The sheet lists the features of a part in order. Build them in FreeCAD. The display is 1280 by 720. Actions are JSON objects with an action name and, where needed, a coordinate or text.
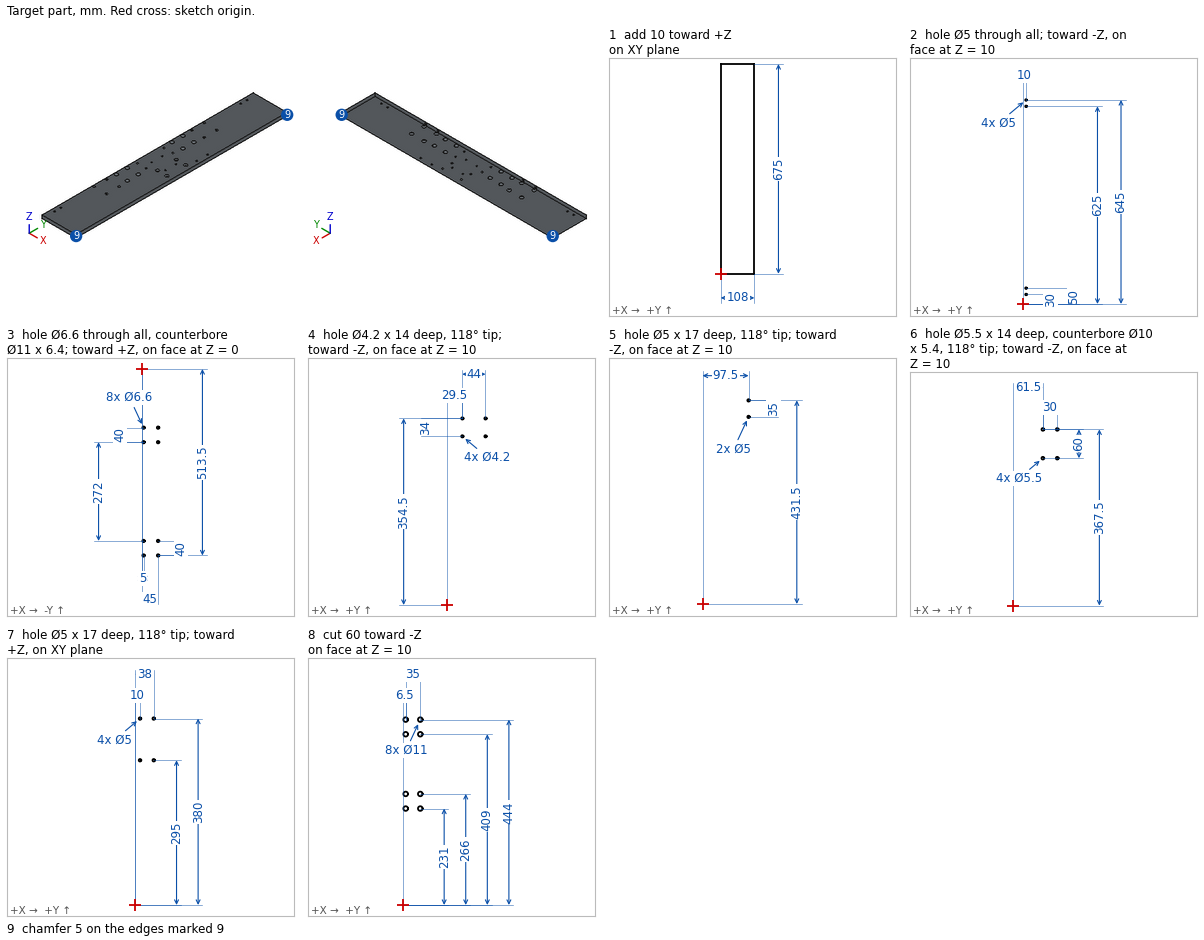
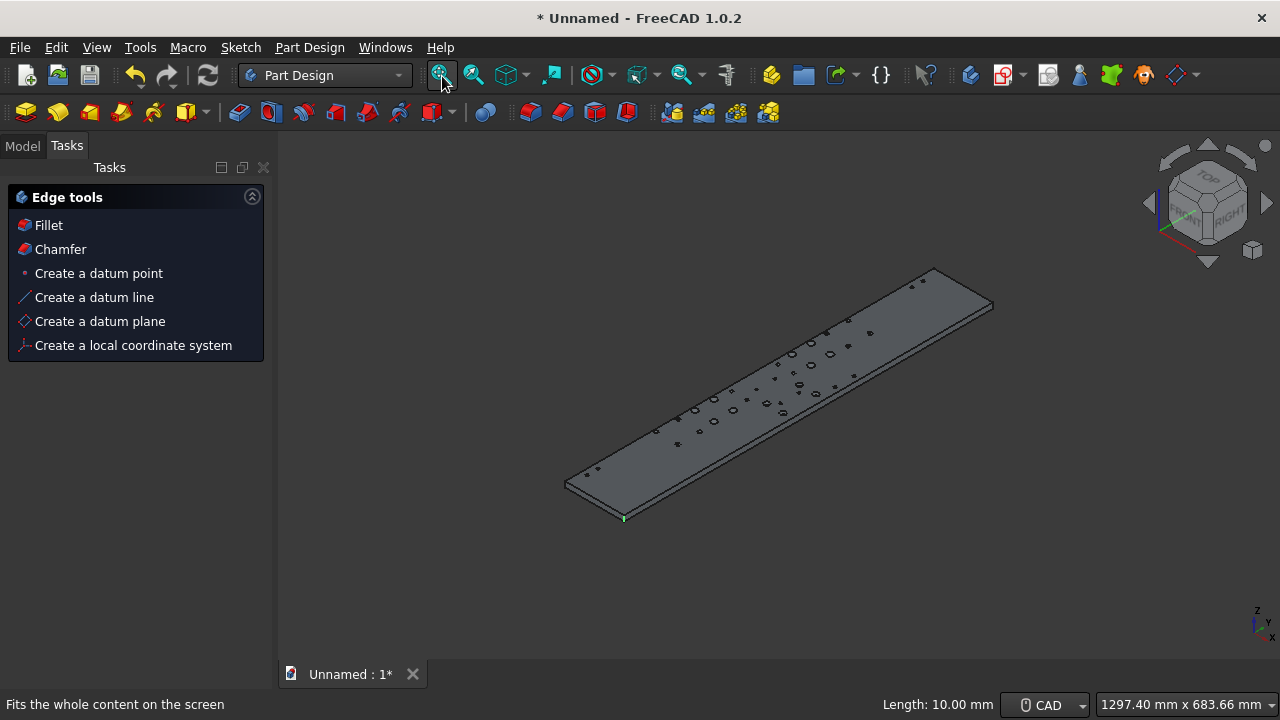
{"action": "scroll", "coordinate": [993, 305], "scroll_direction": "up", "scroll_amount": 9}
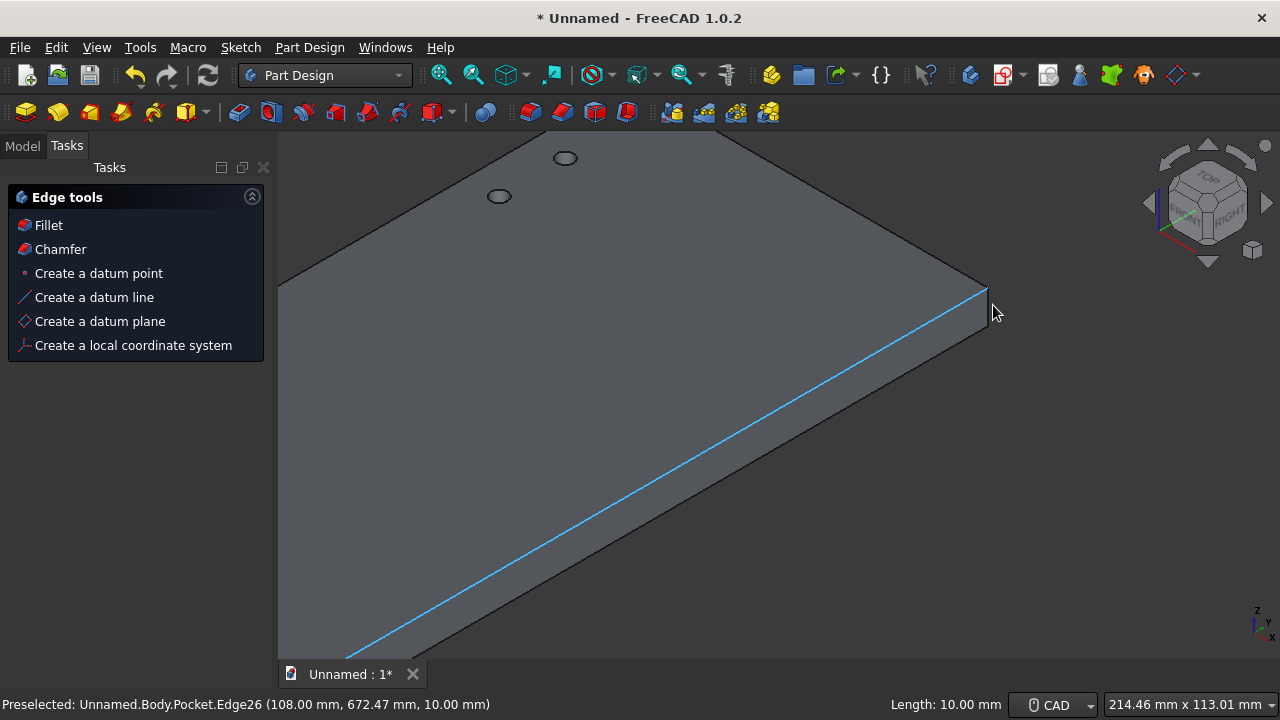
{"action": "left_click", "coordinate": [442, 76]}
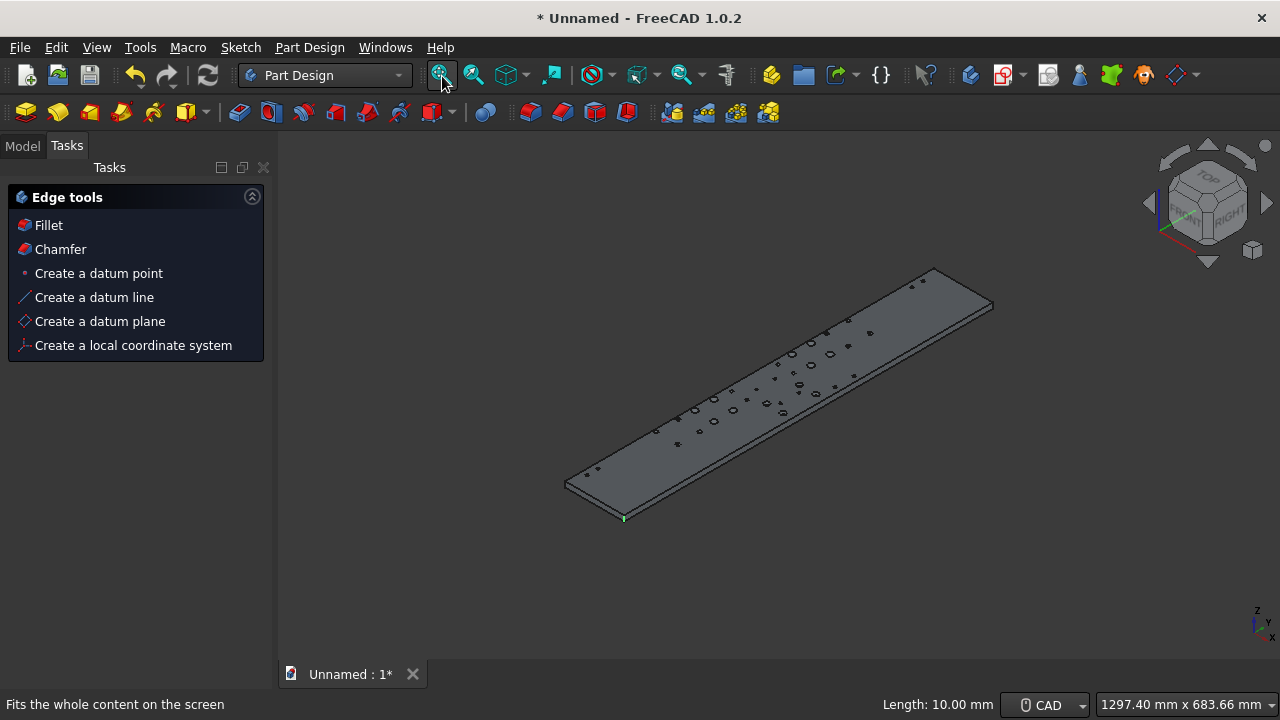
{"action": "key", "text": "1"}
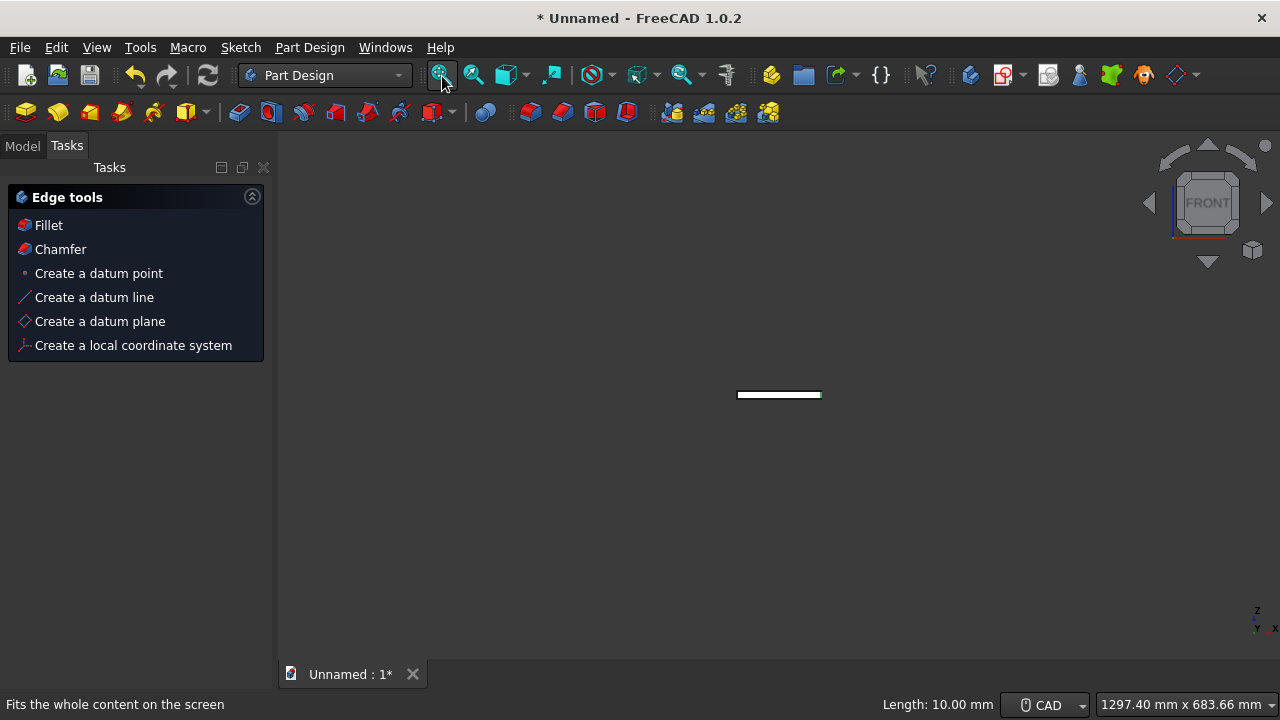
{"action": "left_click", "coordinate": [442, 76]}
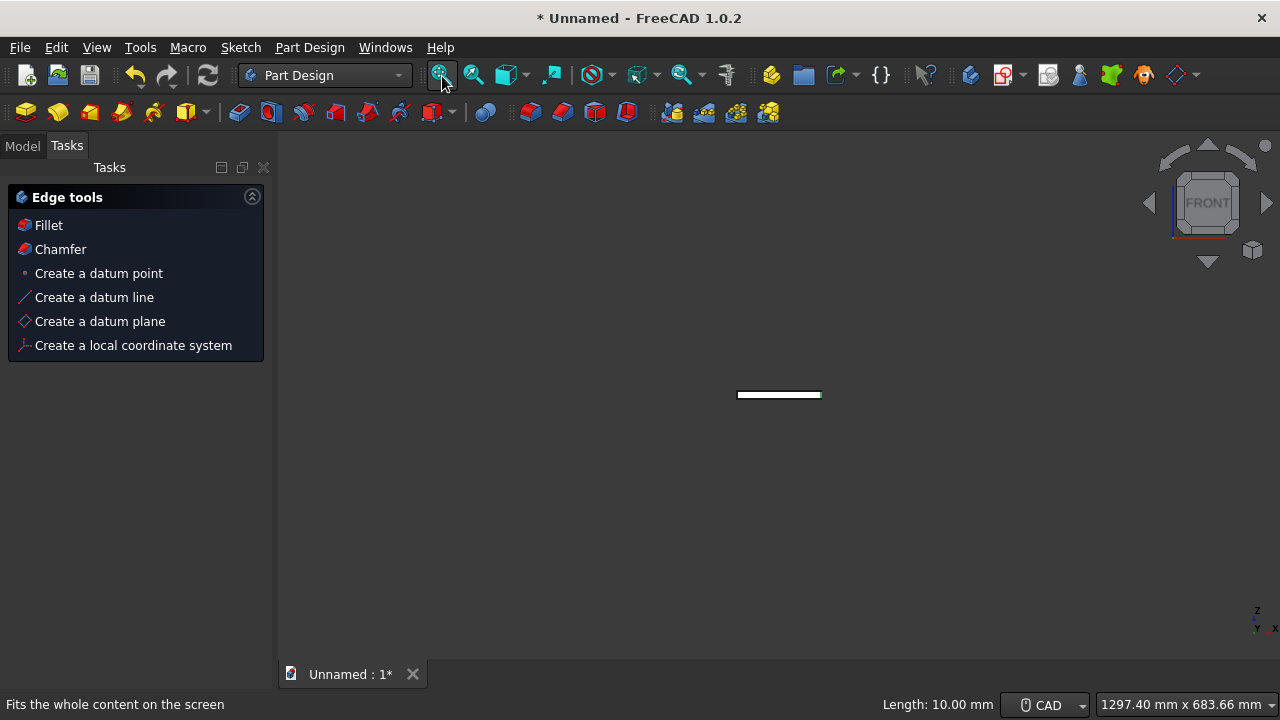
{"action": "scroll", "coordinate": [821, 394], "scroll_direction": "up", "scroll_amount": 9}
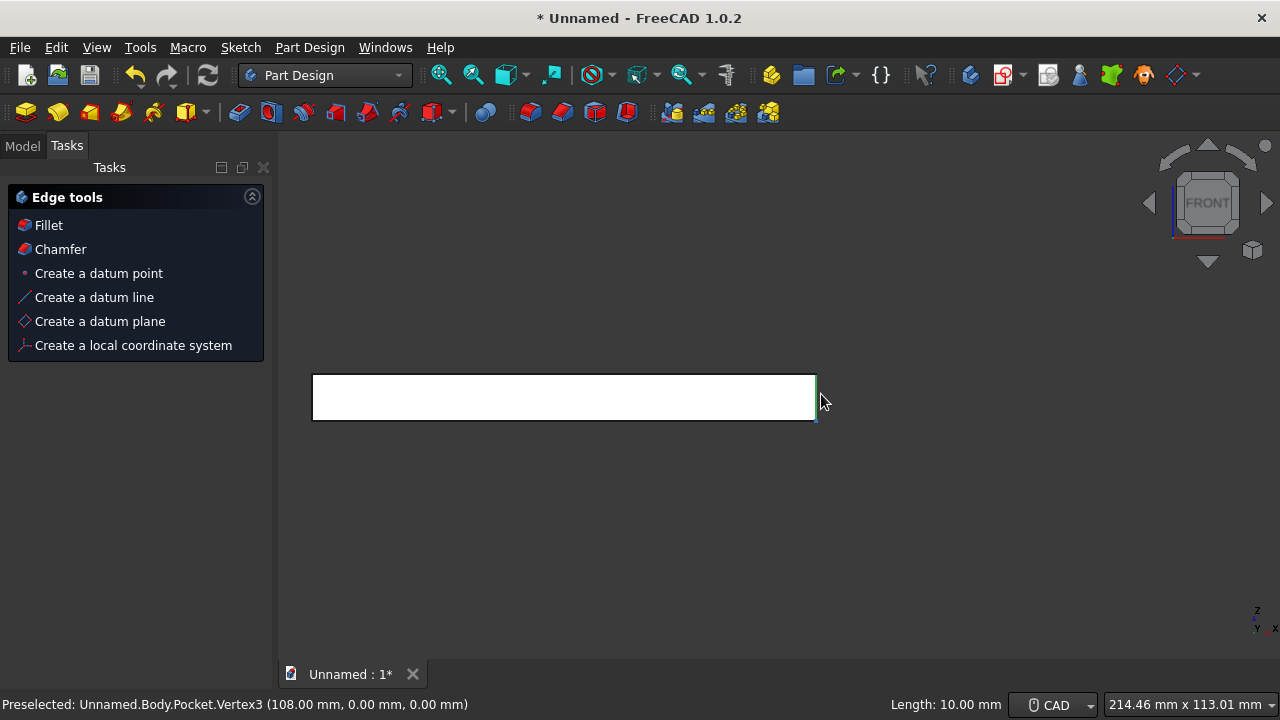
{"action": "left_click", "coordinate": [442, 76]}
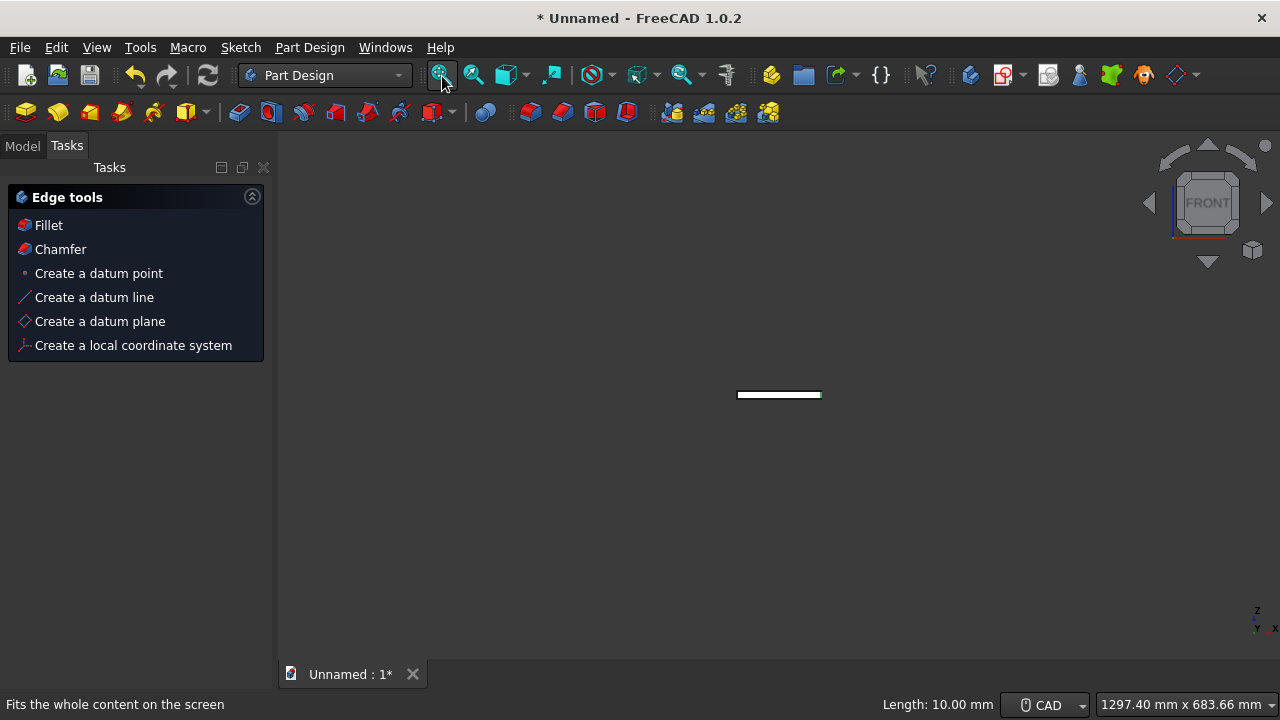
{"action": "key", "text": "3"}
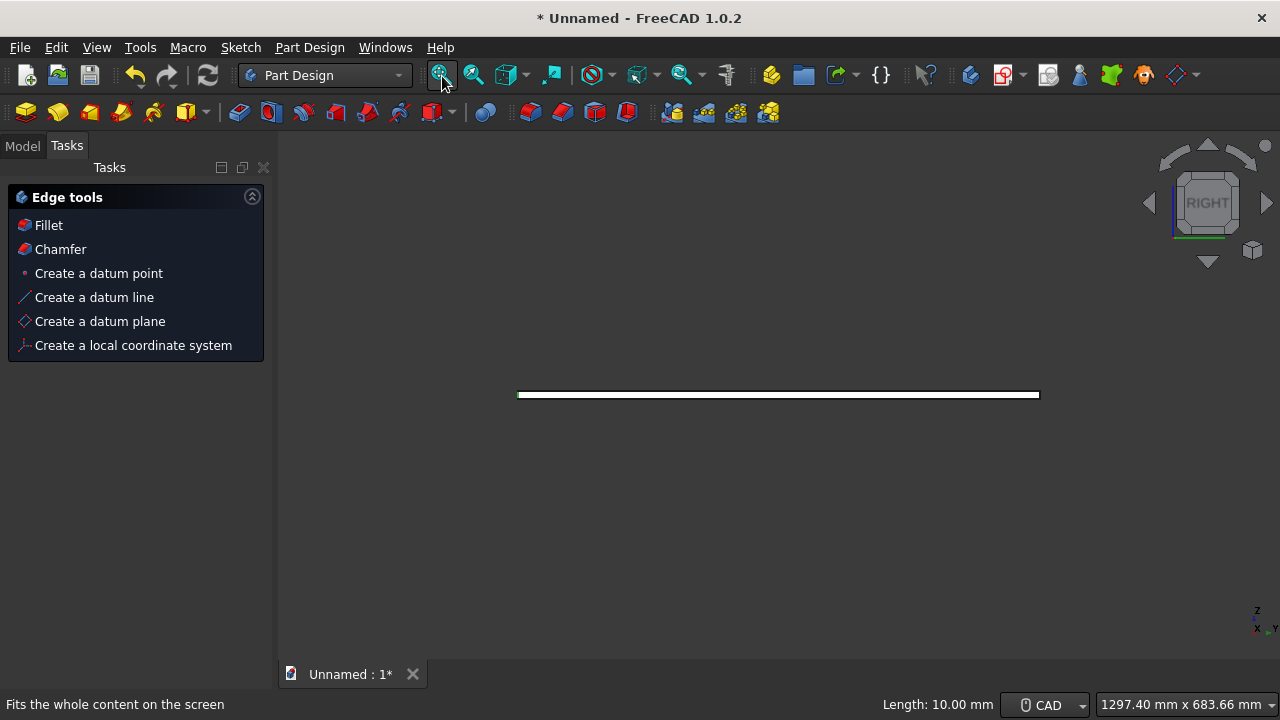
{"action": "scroll", "coordinate": [1040, 394], "scroll_direction": "up", "scroll_amount": 9}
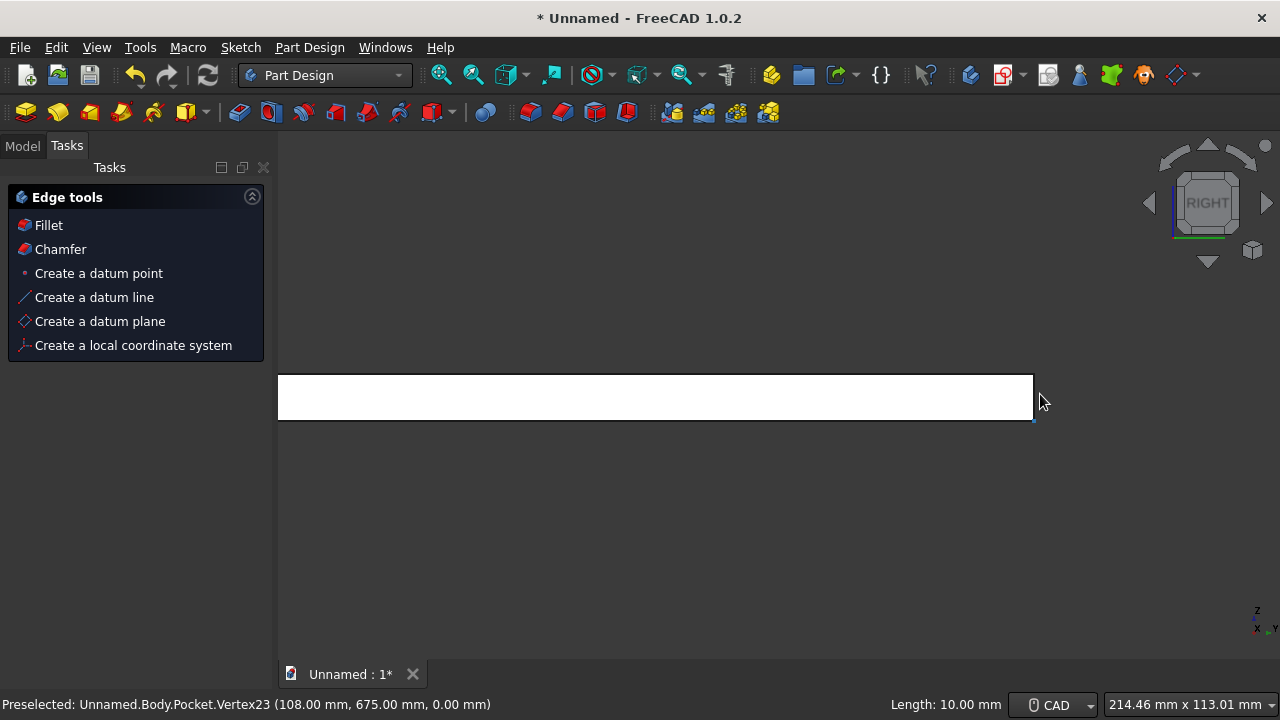
{"action": "left_click", "coordinate": [1034, 397], "text": "ctrl"}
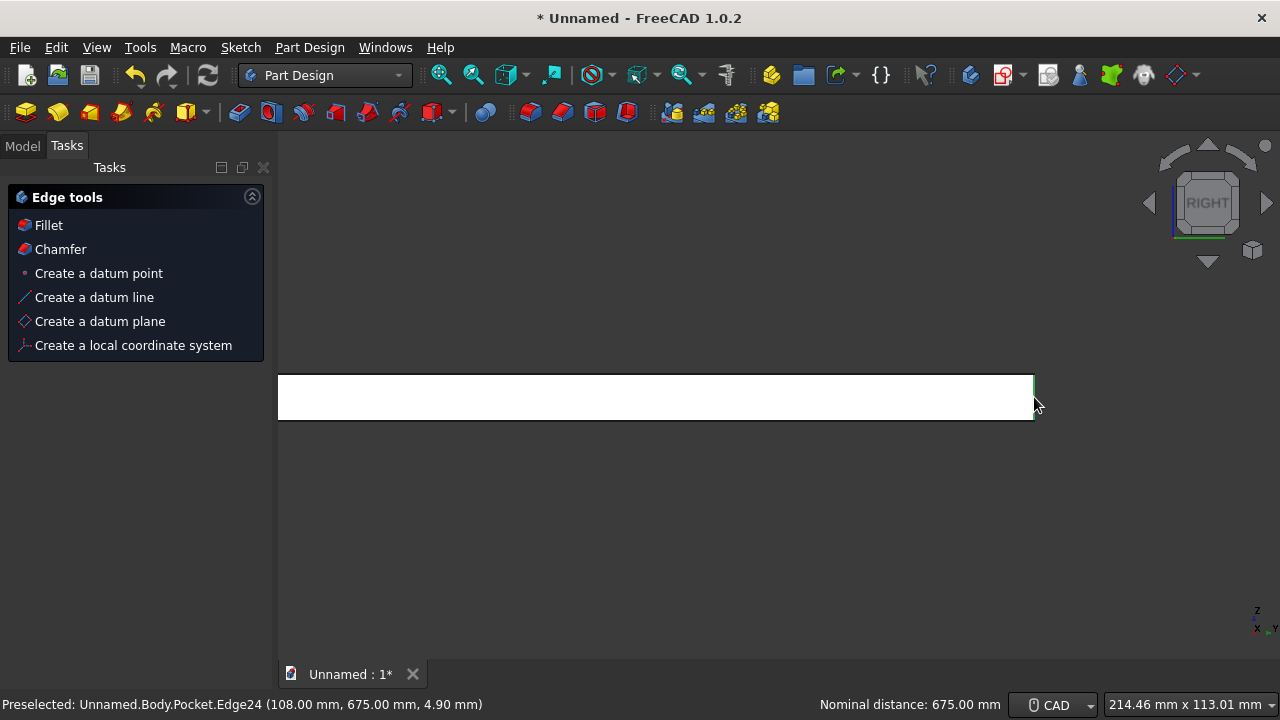
{"action": "left_click", "coordinate": [564, 112]}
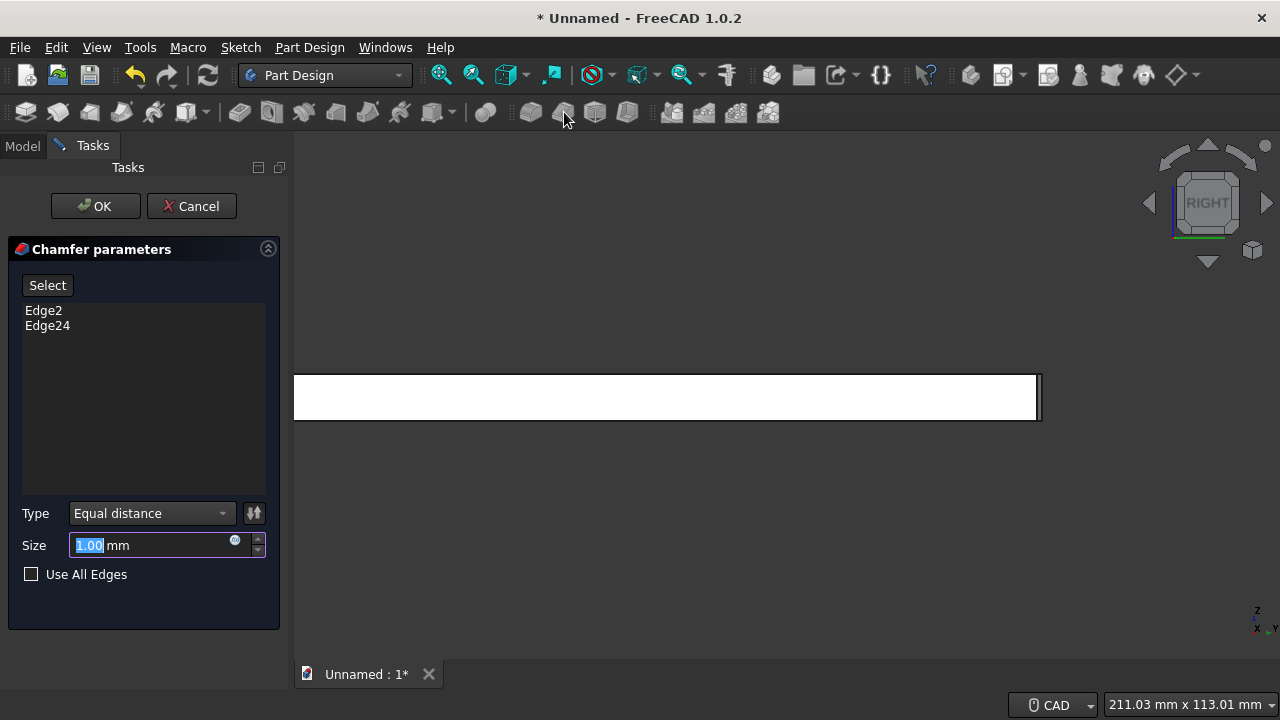
{"action": "type", "text": "5"}
{"action": "key", "text": "Tab"}